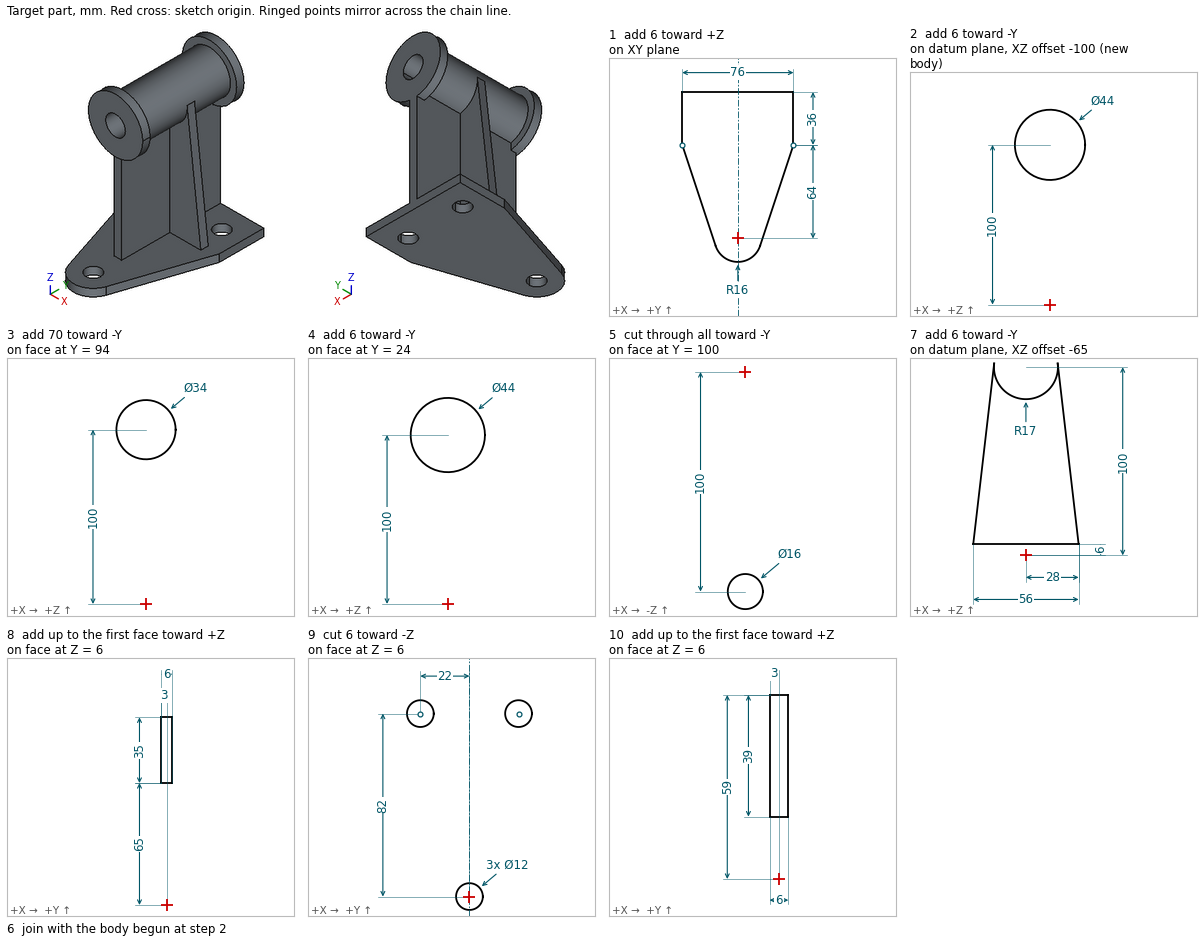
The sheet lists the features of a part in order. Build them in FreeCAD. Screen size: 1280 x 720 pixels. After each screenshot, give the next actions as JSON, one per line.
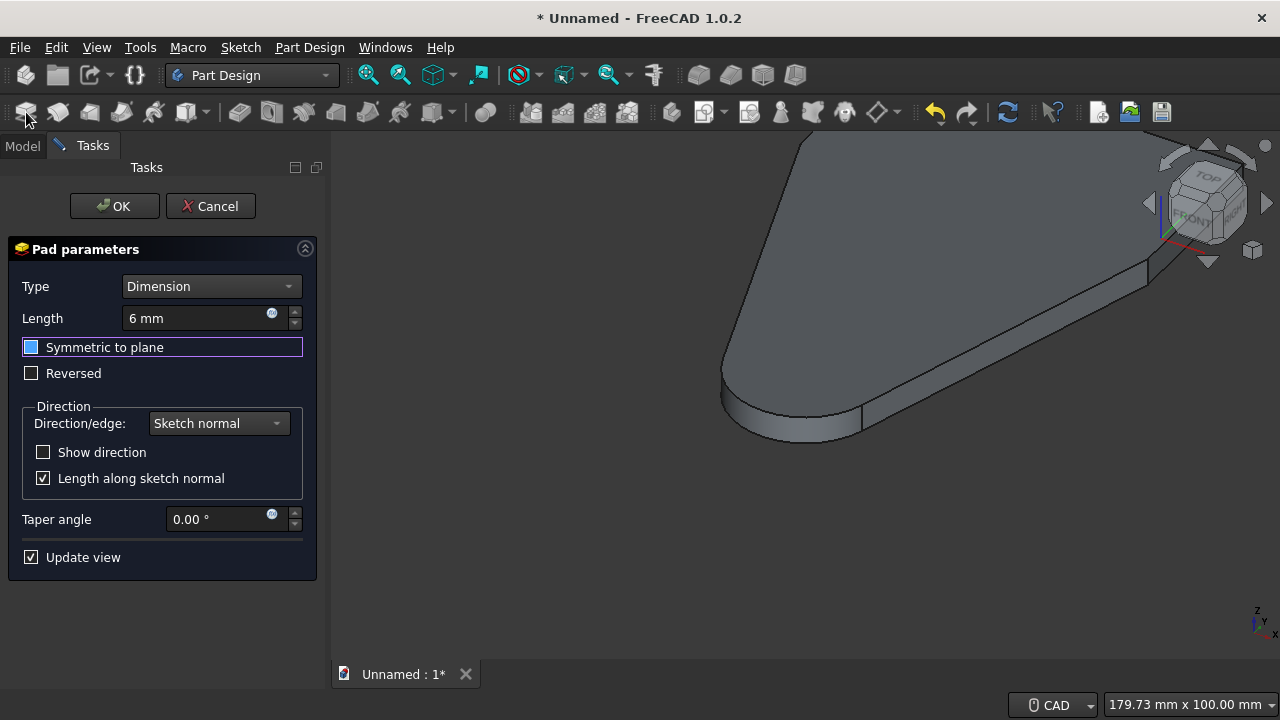
{"action": "left_click", "coordinate": [115, 206]}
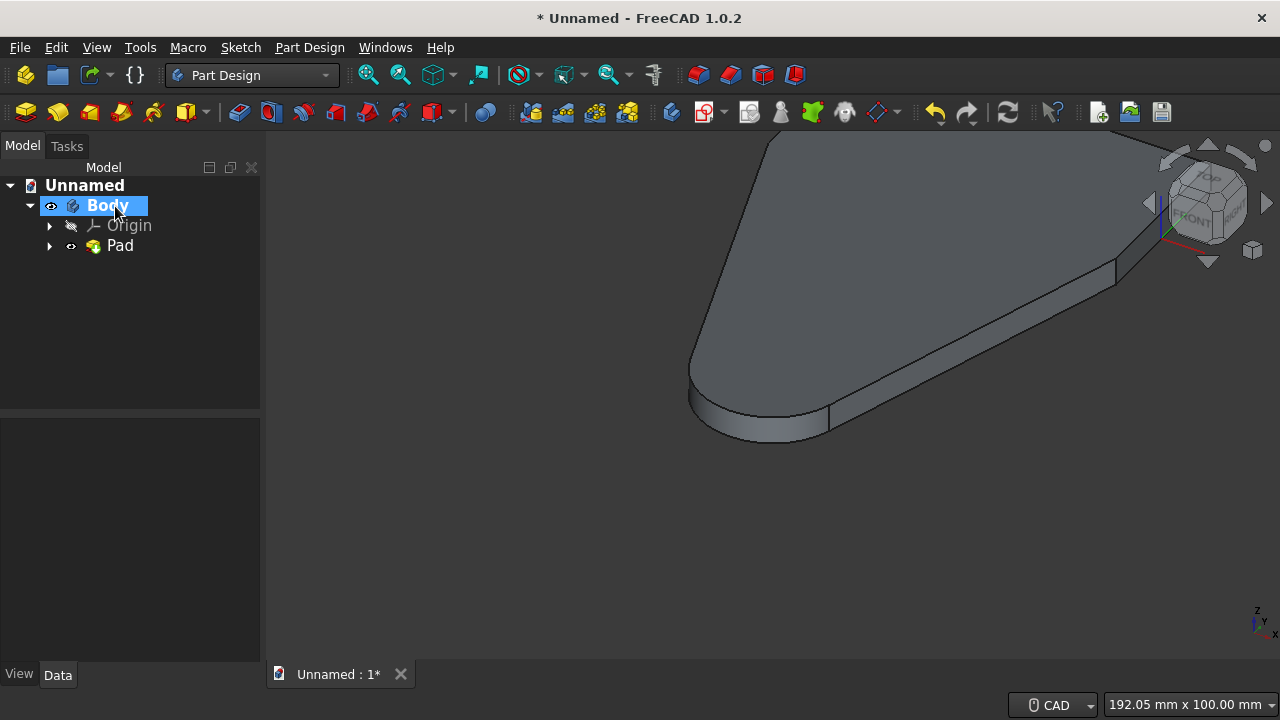
{"action": "key", "text": "v f"}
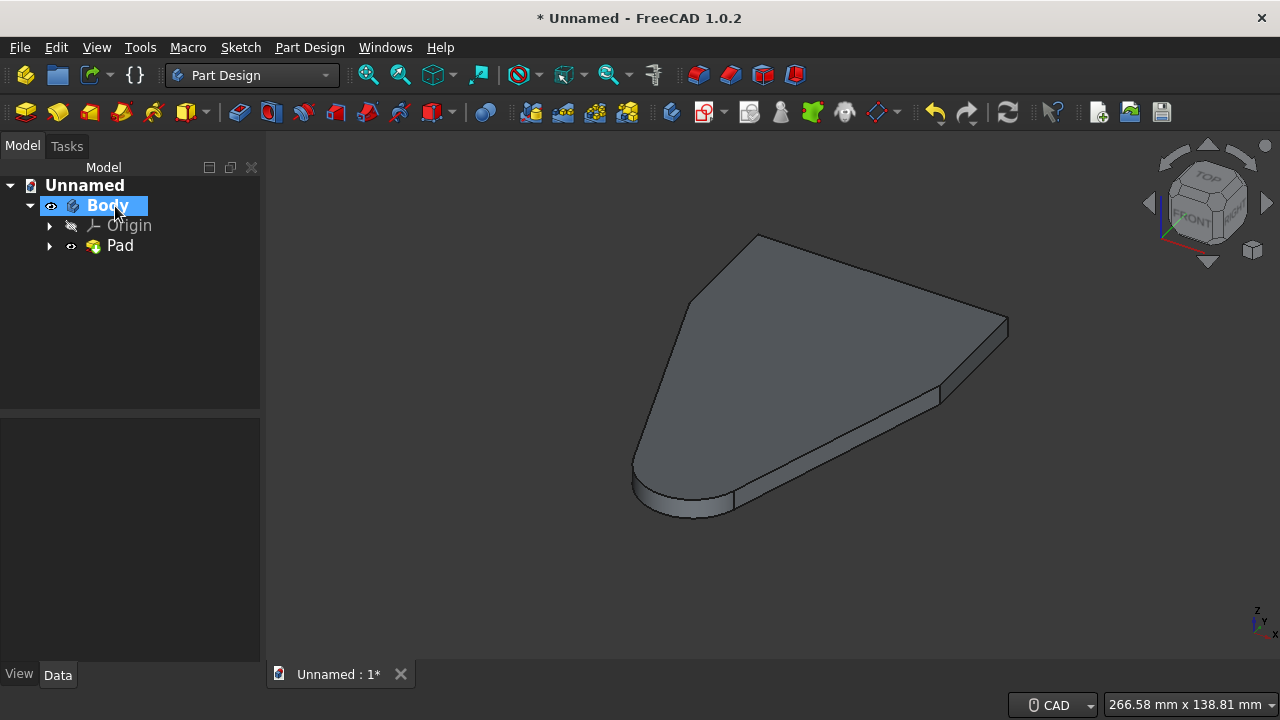
{"action": "left_click", "coordinate": [672, 112]}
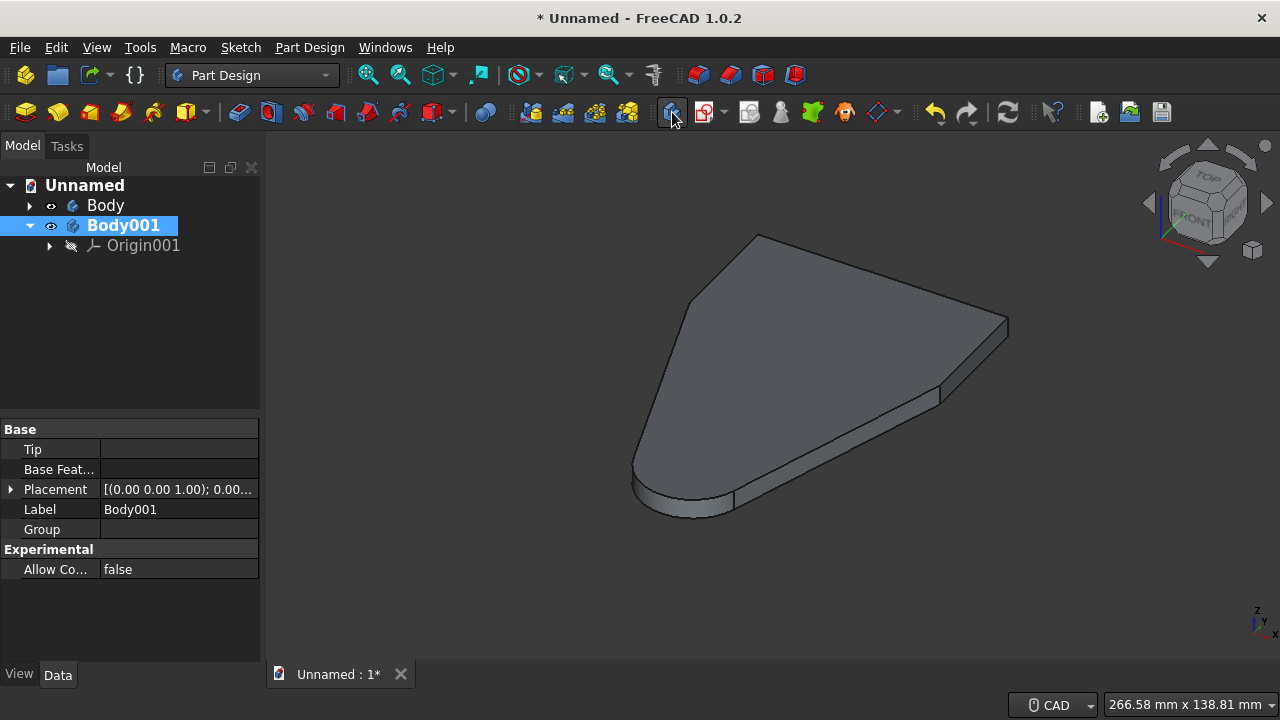
{"action": "left_click", "coordinate": [50, 246]}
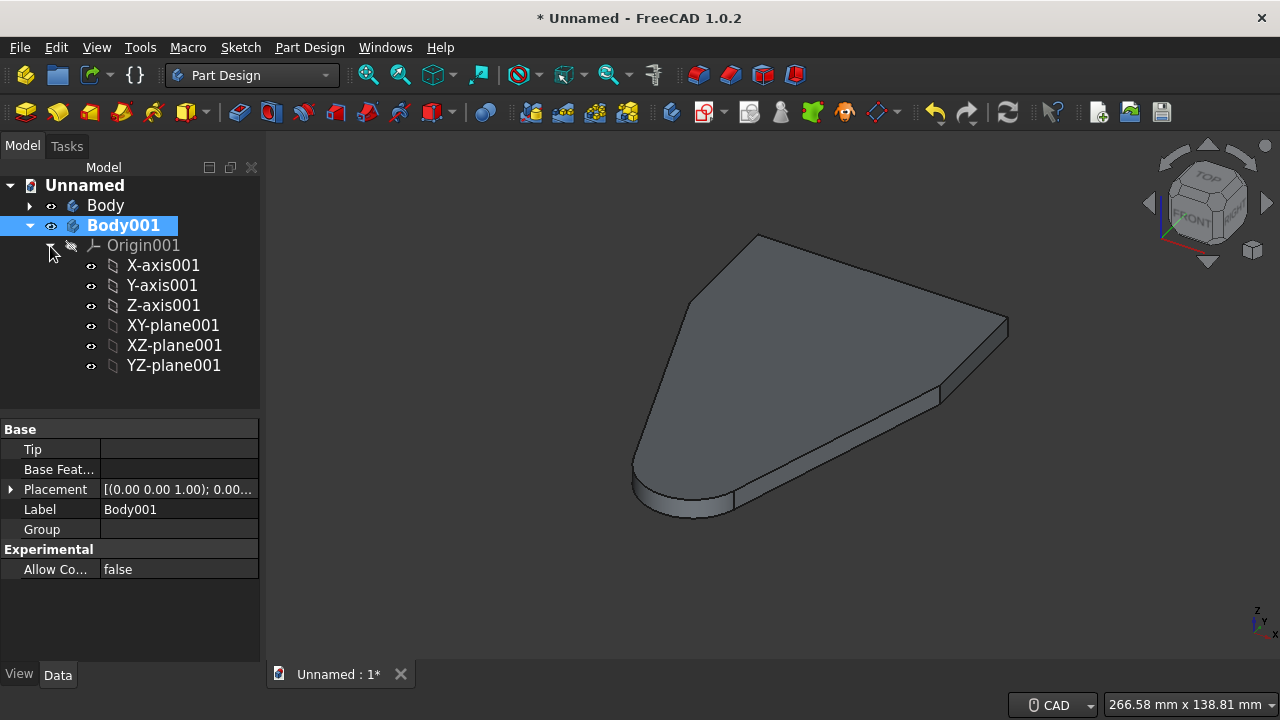
{"action": "left_click", "coordinate": [136, 346]}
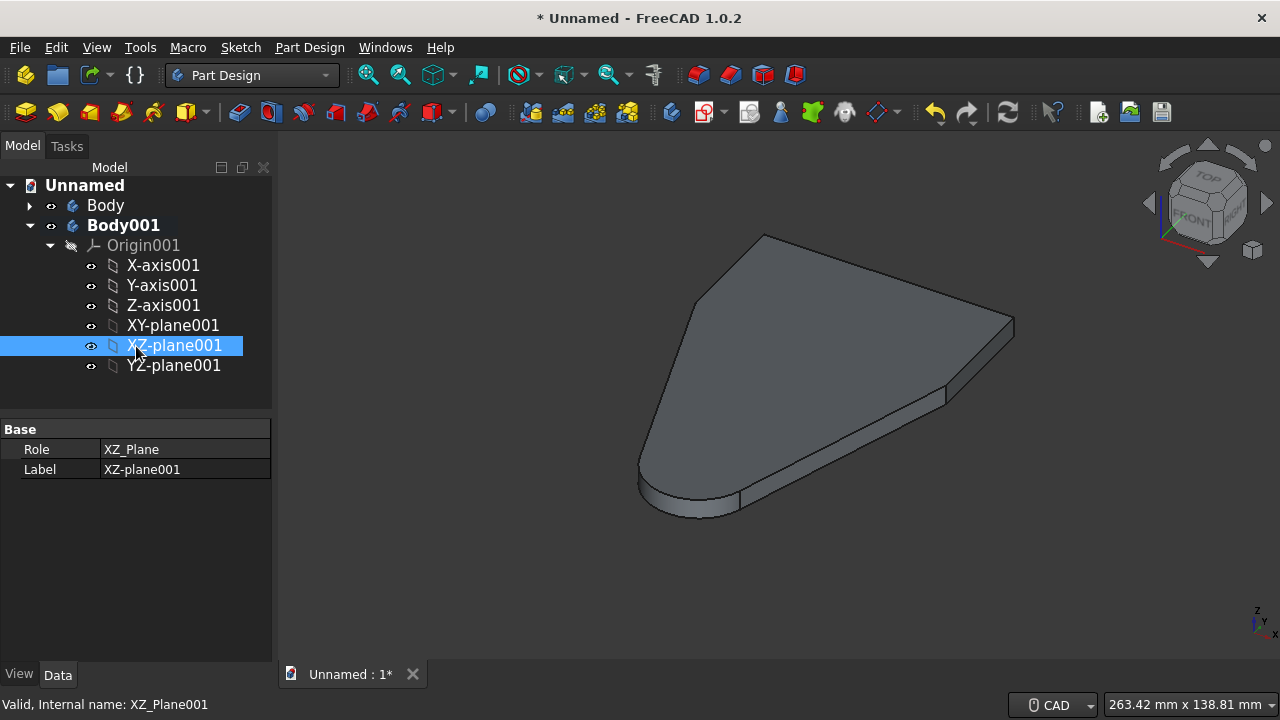
{"action": "left_click", "coordinate": [878, 112]}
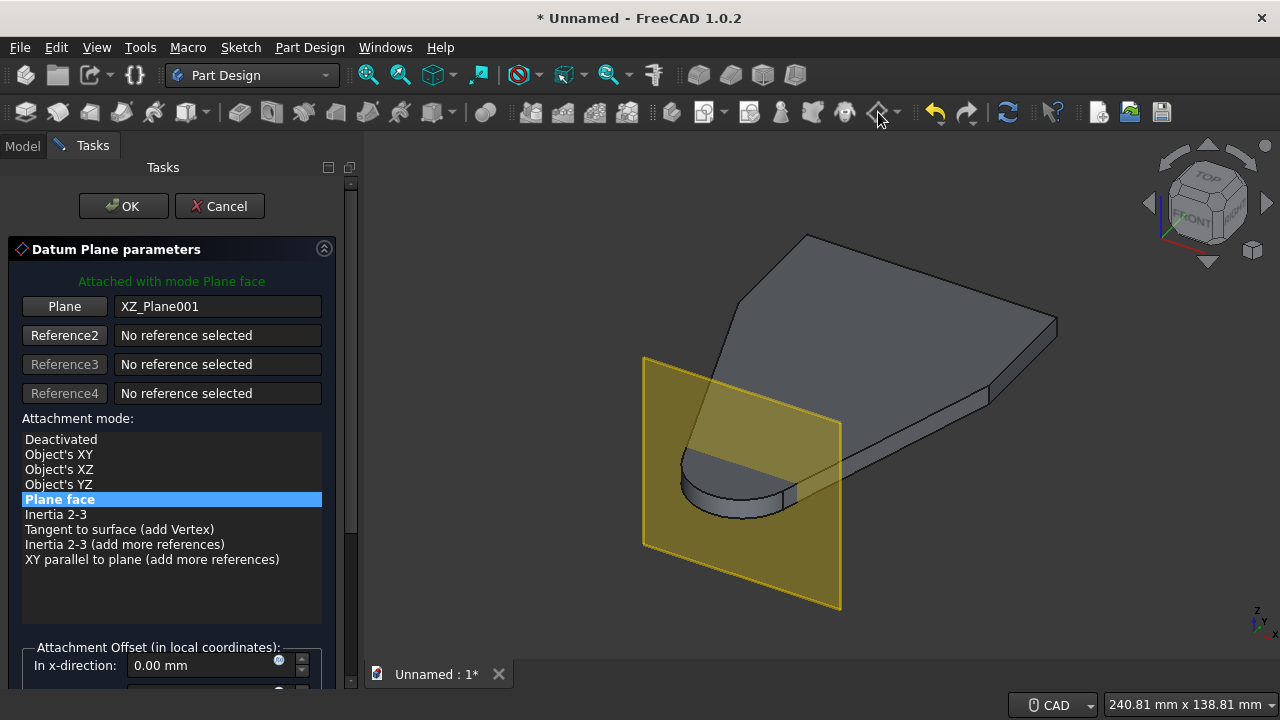
{"action": "scroll", "coordinate": [351, 432], "scroll_direction": "down", "scroll_amount": 2}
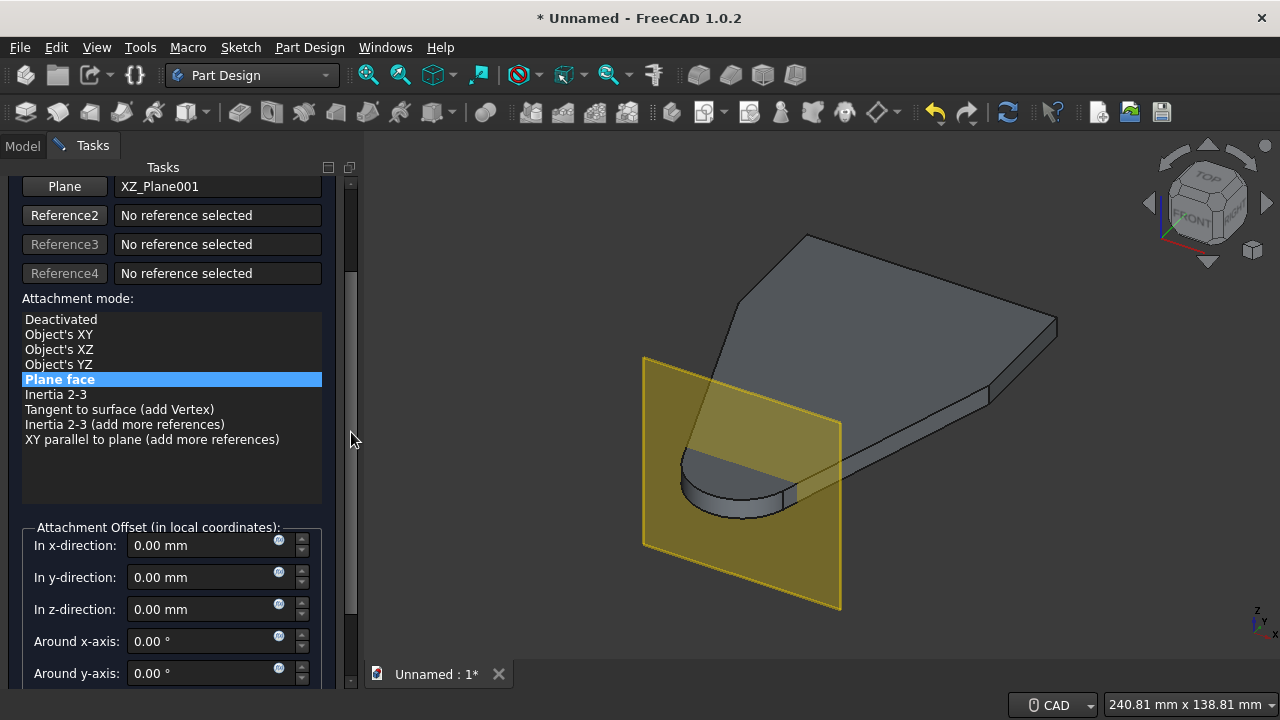
{"action": "triple_click", "coordinate": [210, 609]}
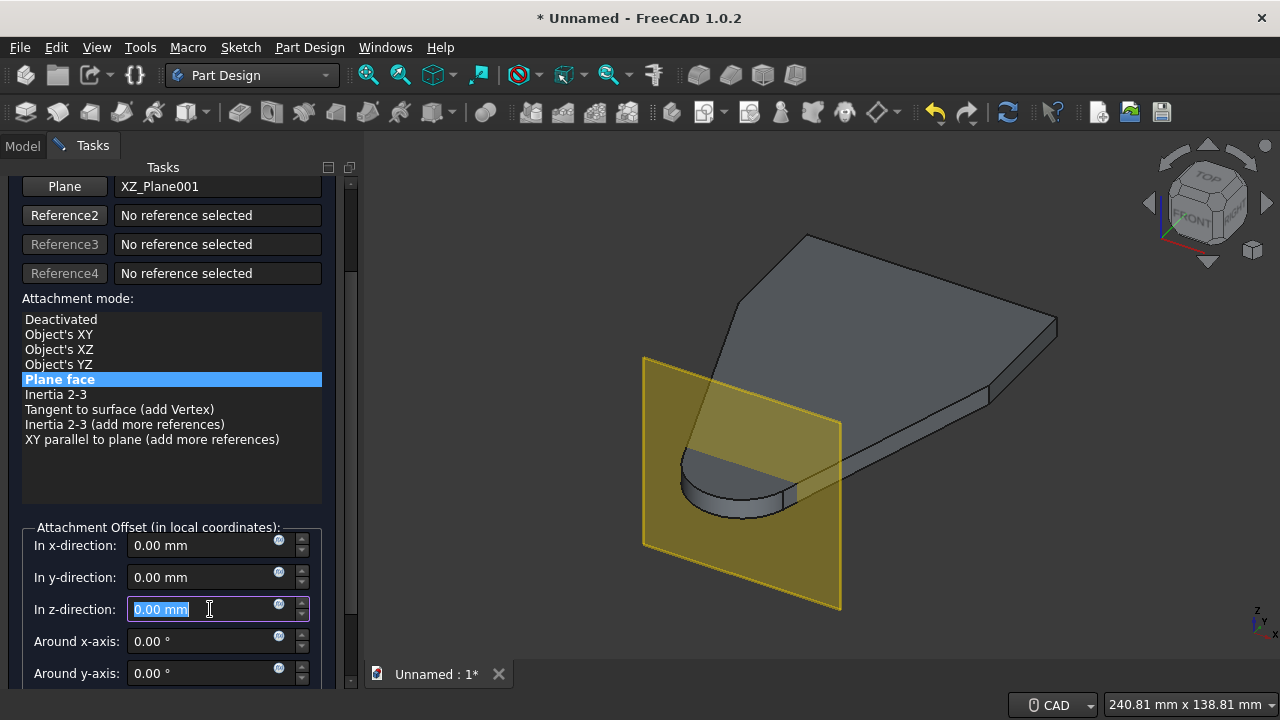
{"action": "type", "text": "-100"}
{"action": "key", "text": "Tab"}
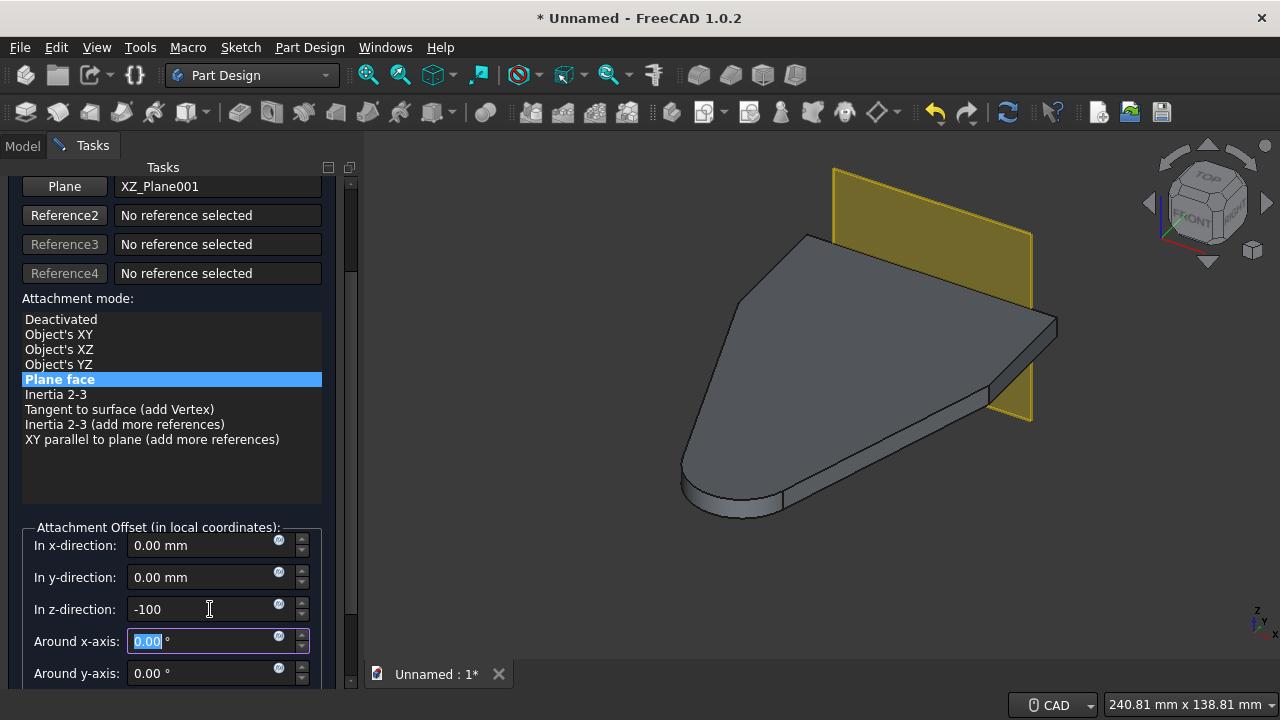
{"action": "scroll", "coordinate": [351, 432], "scroll_direction": "up", "scroll_amount": 3}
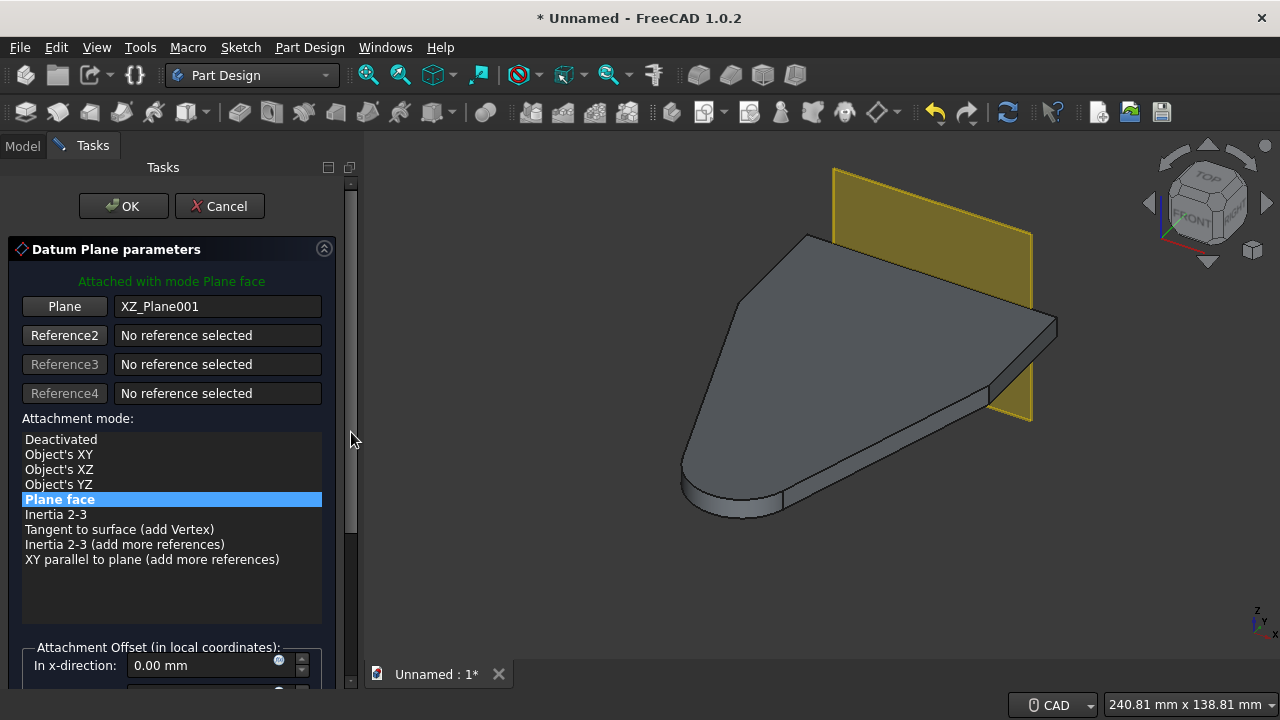
{"action": "left_click", "coordinate": [124, 206]}